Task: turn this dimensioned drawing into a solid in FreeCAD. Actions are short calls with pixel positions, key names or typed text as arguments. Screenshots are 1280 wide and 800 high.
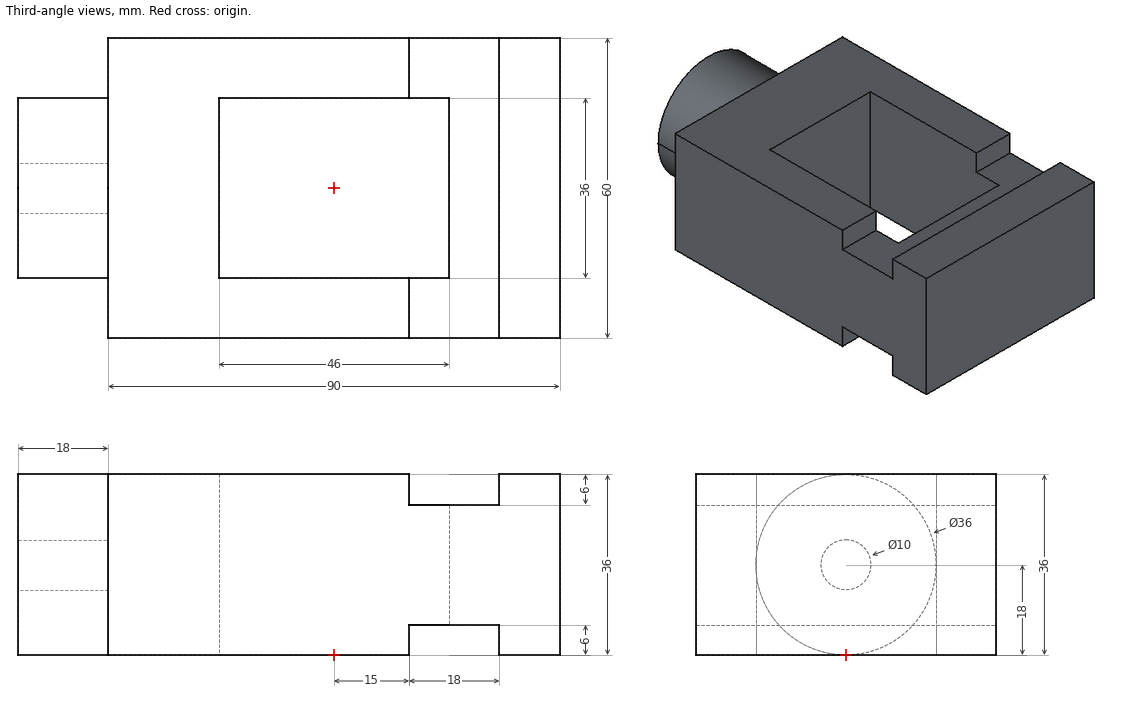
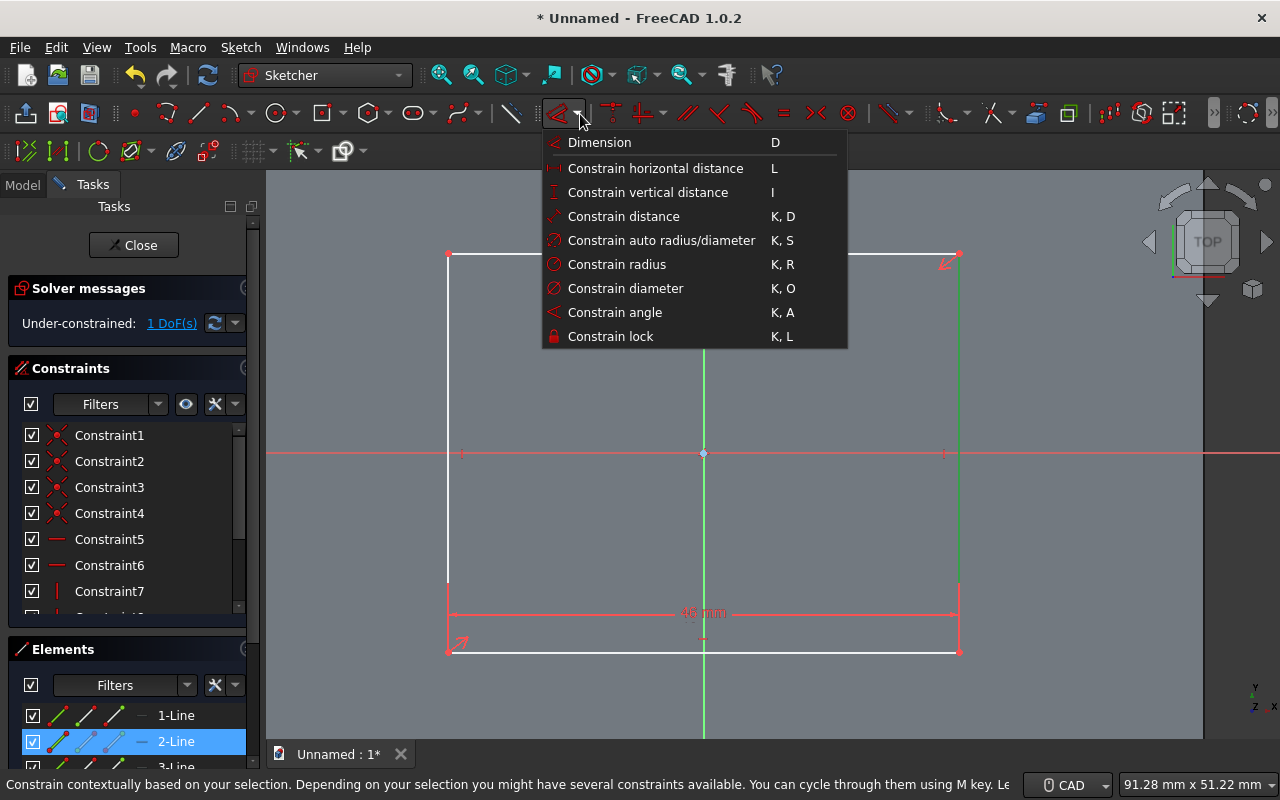
click(695, 192)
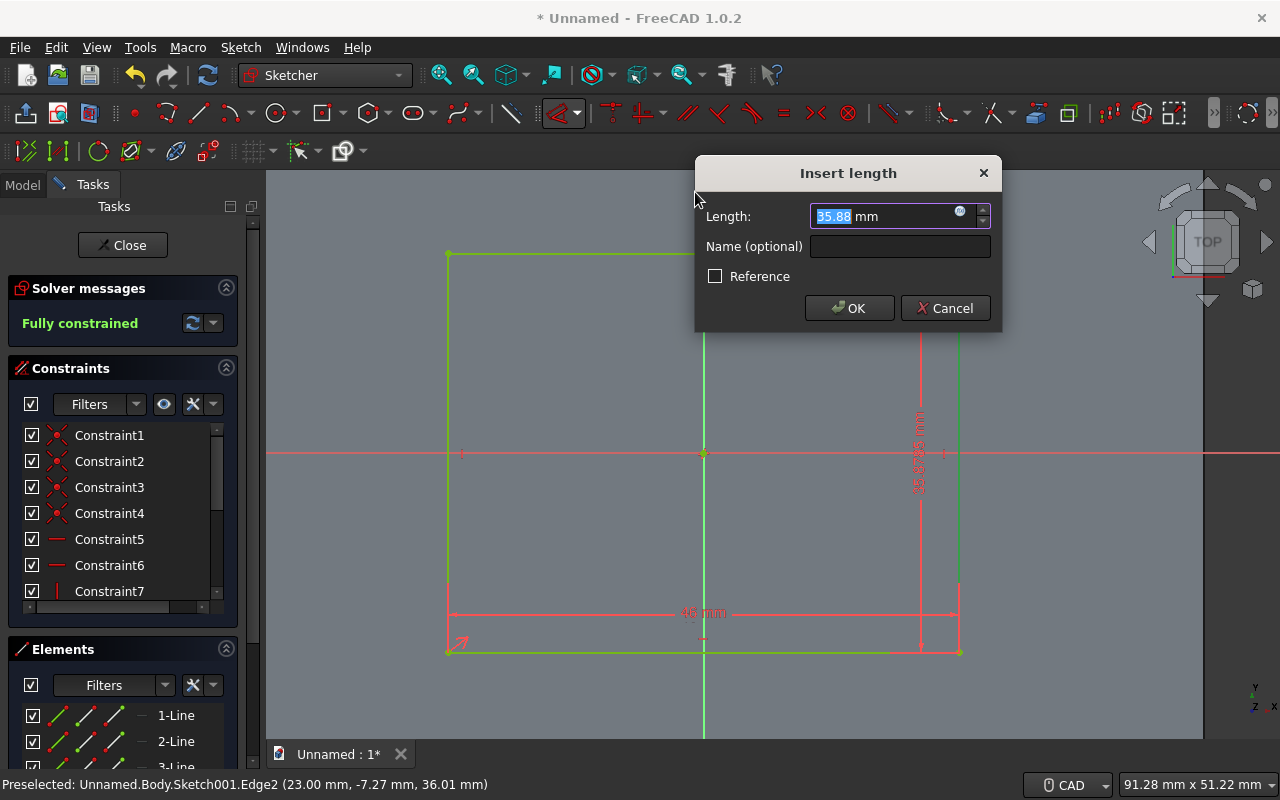
text(36)
key(Return)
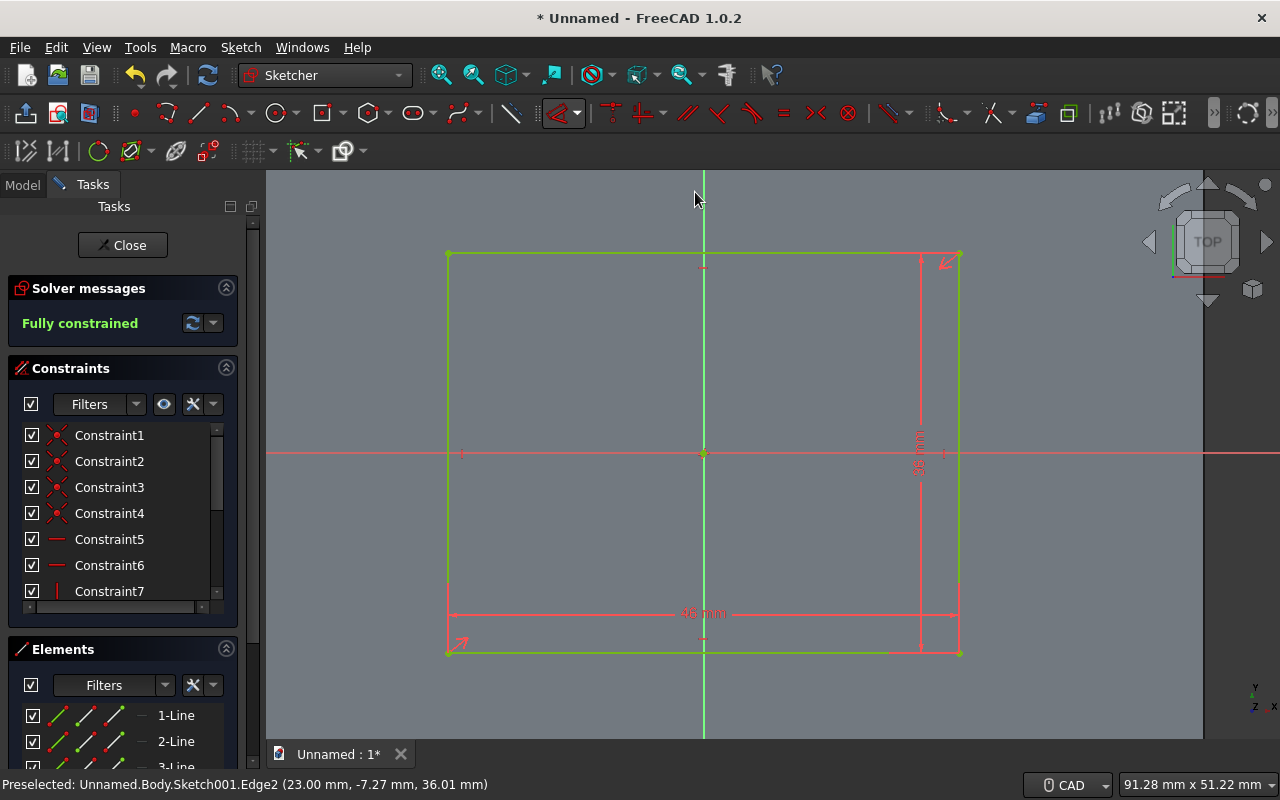
click(123, 245)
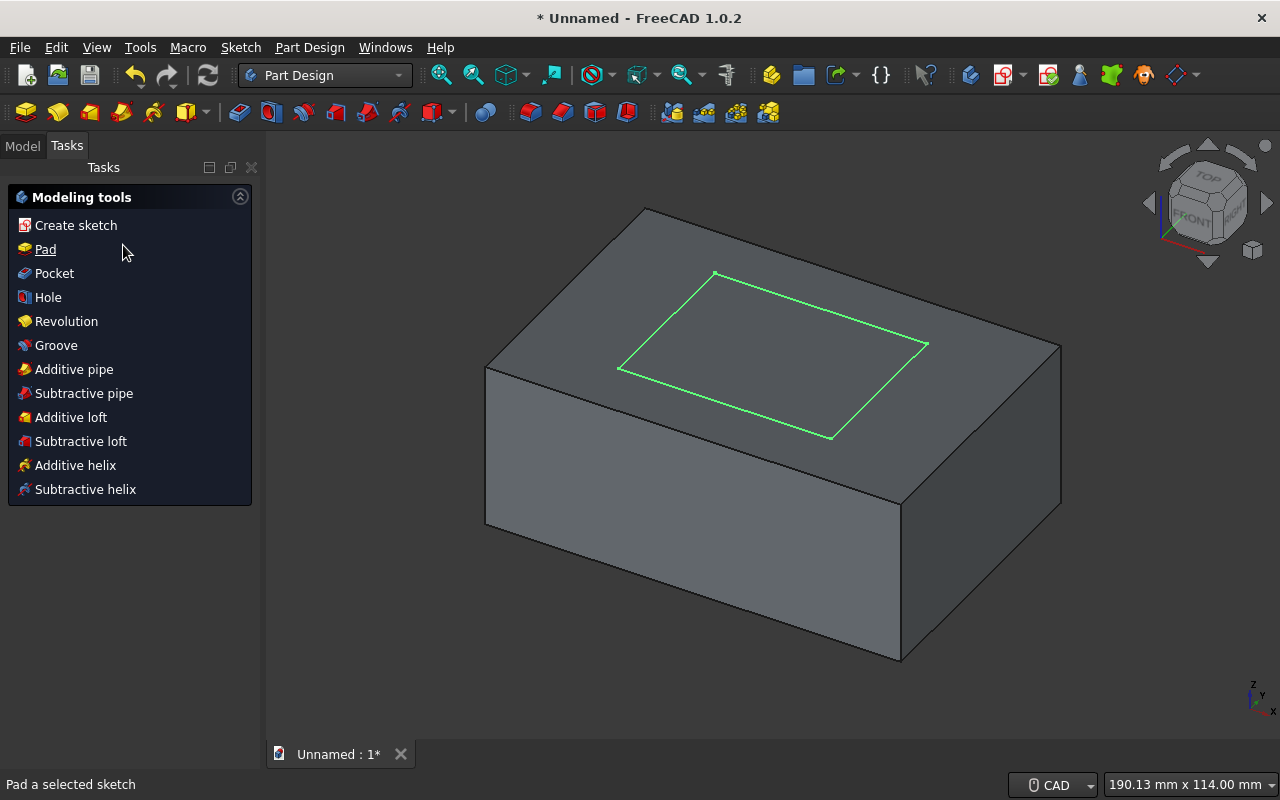
click(240, 112)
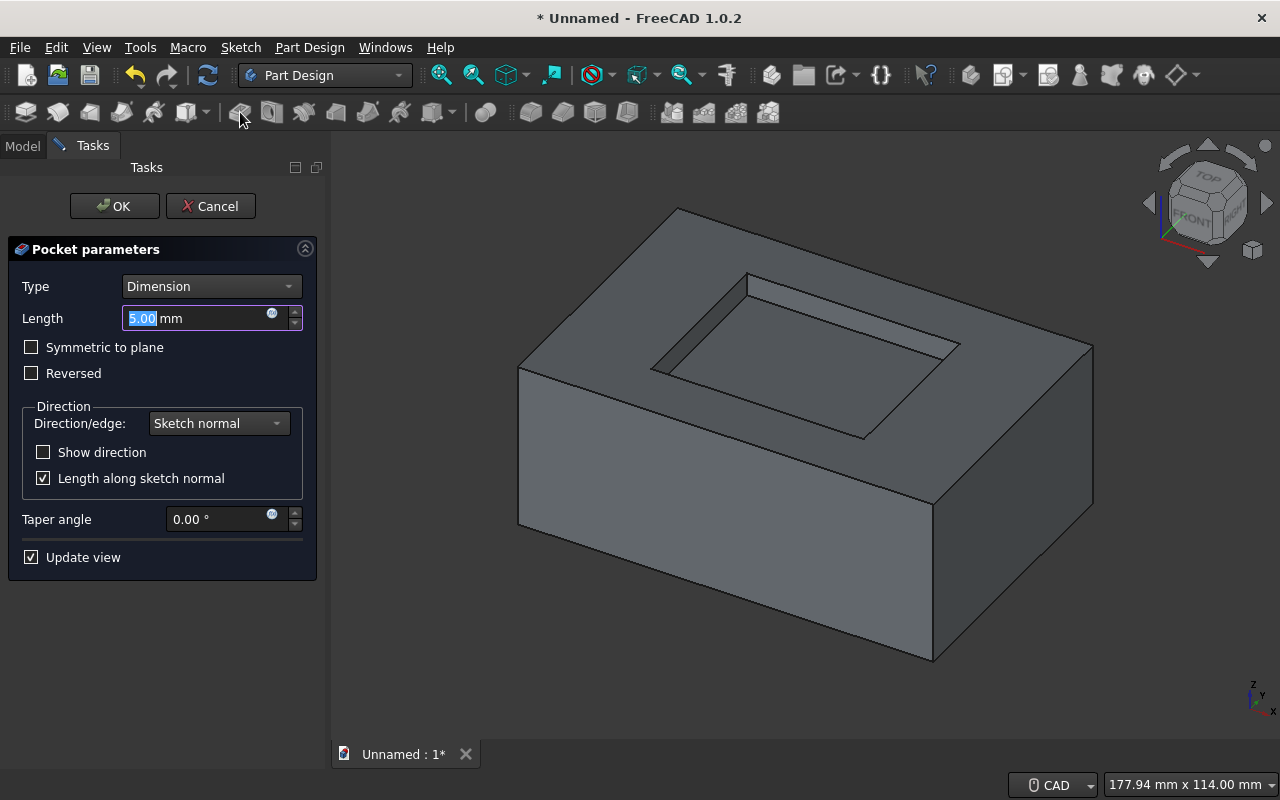
text(36)
key(Tab)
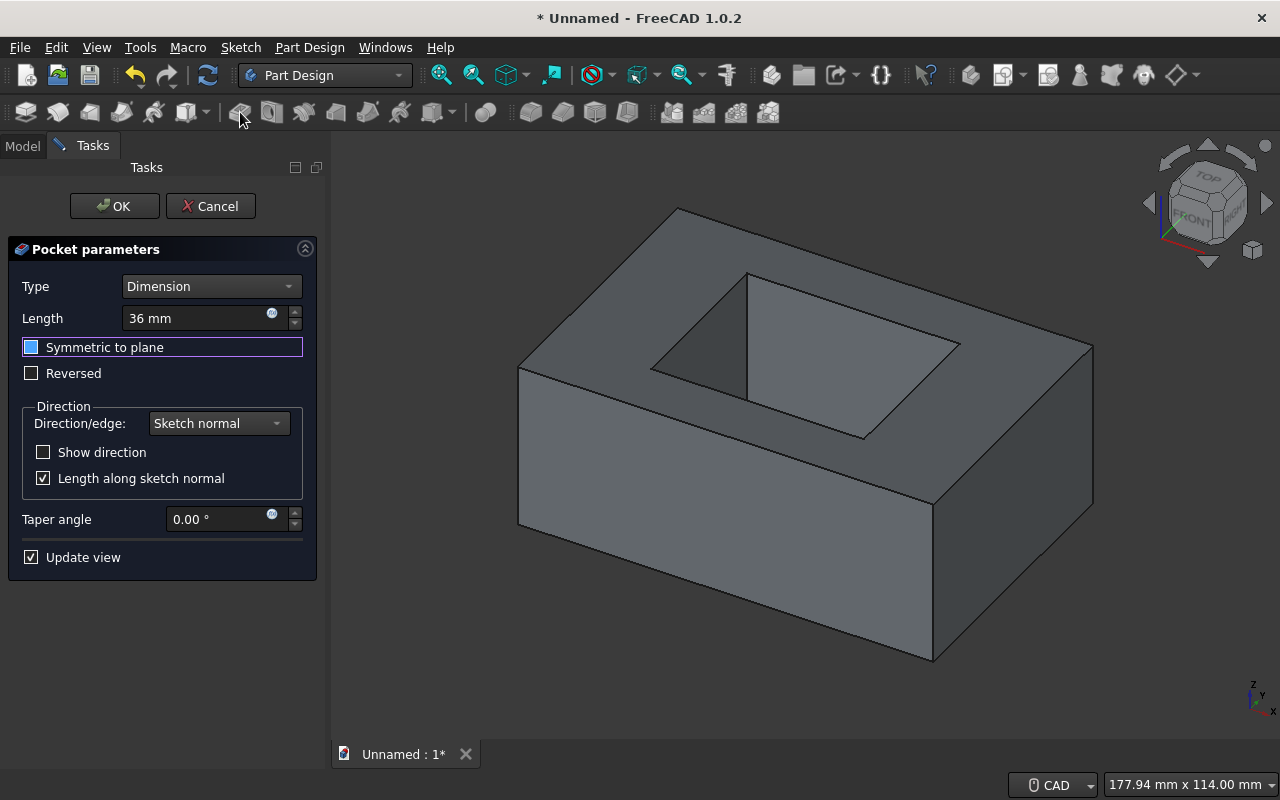
click(115, 206)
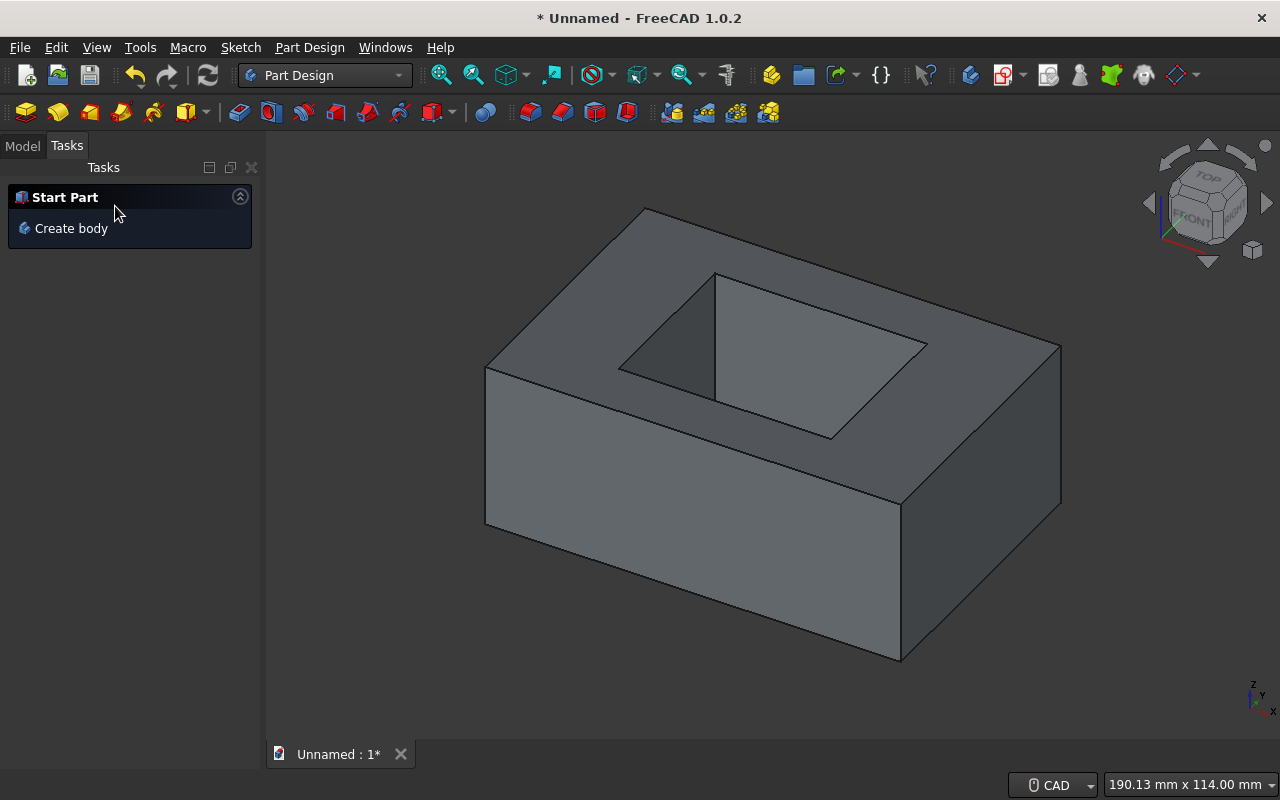
key(6)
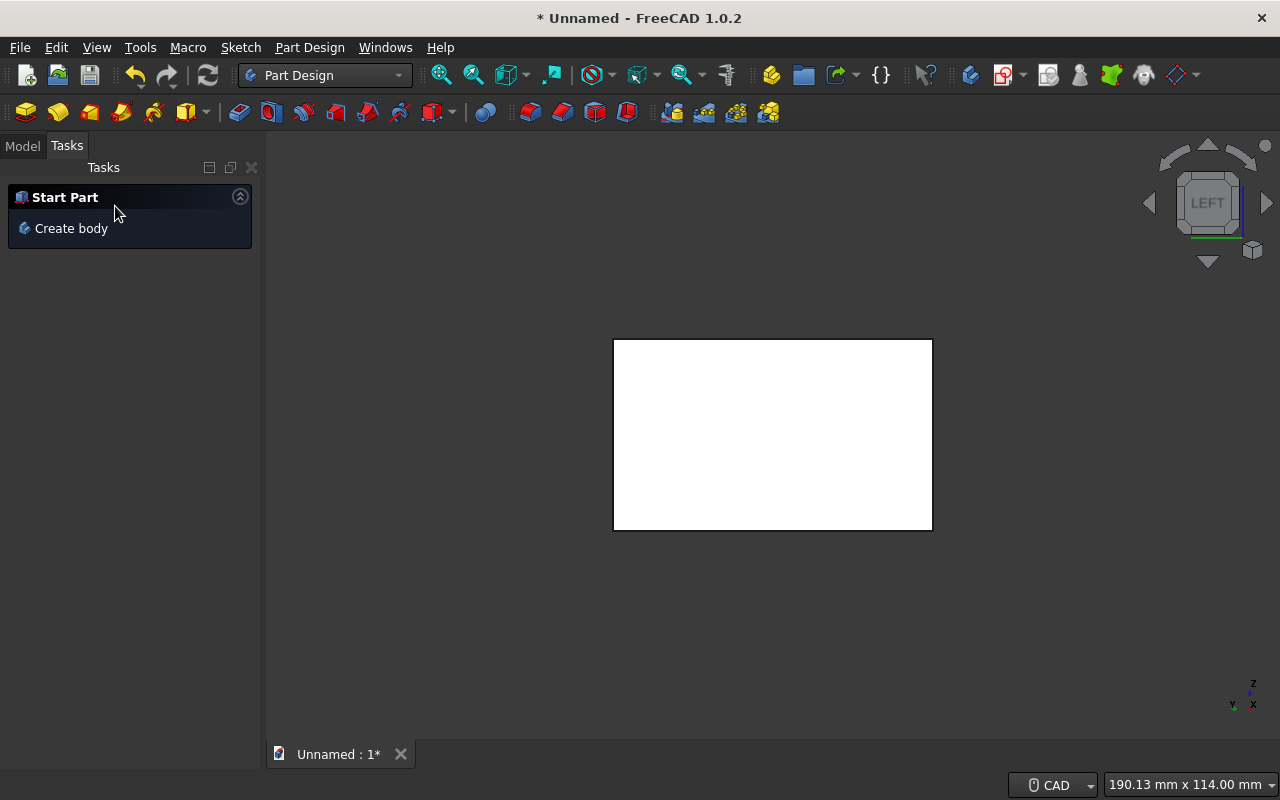
click(442, 76)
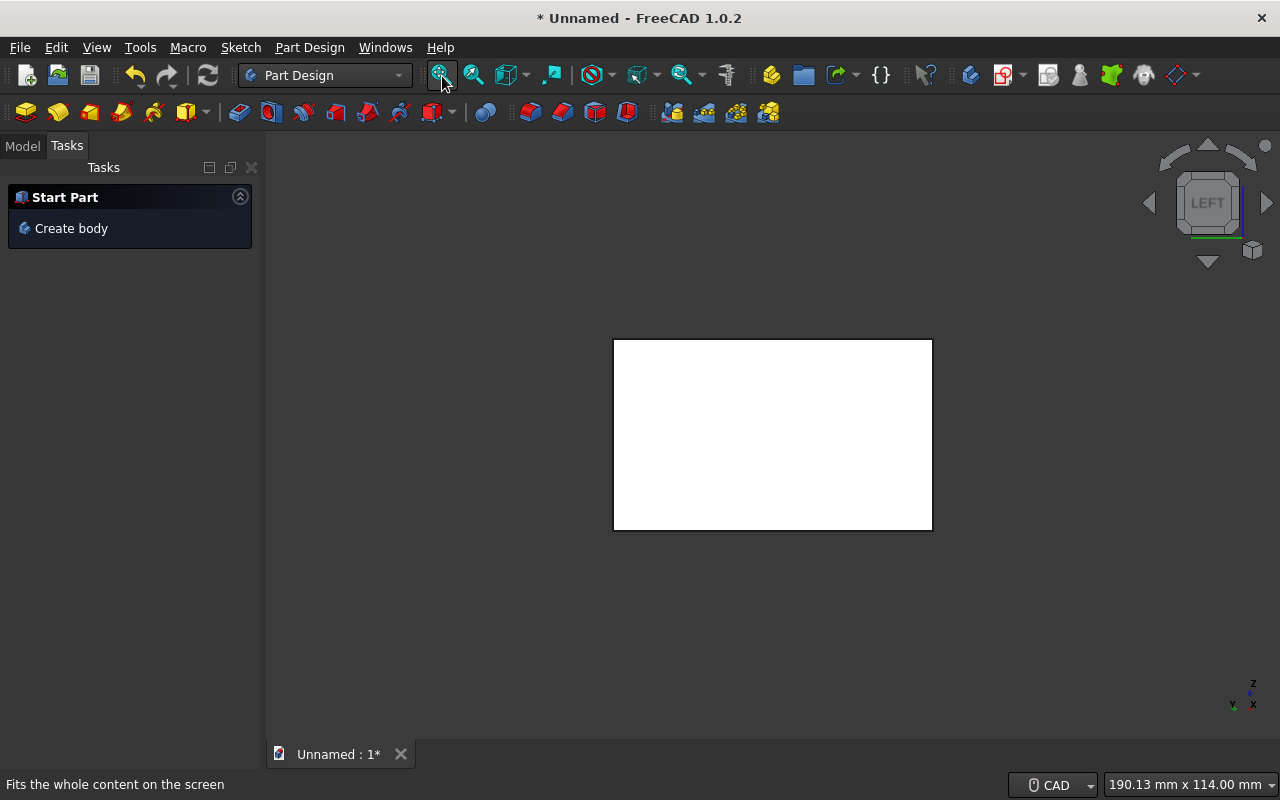
click(727, 434)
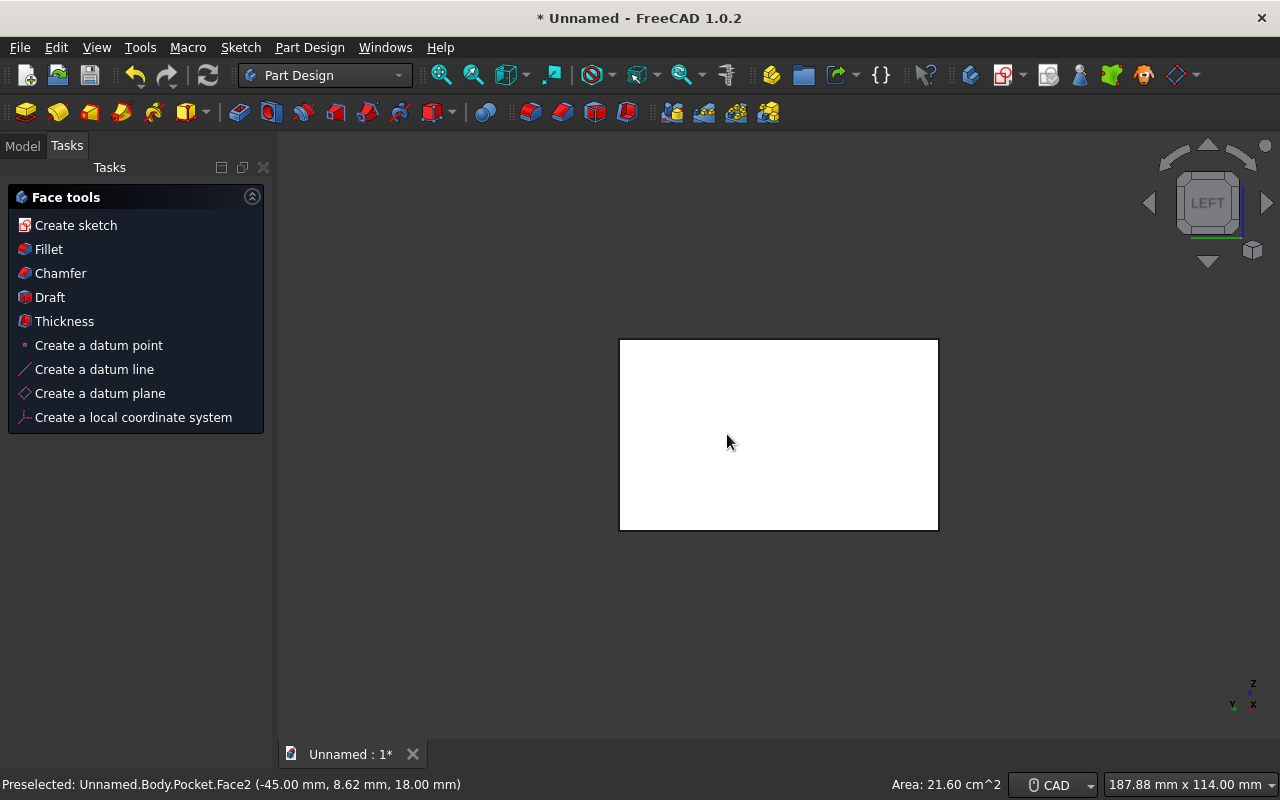
click(1004, 76)